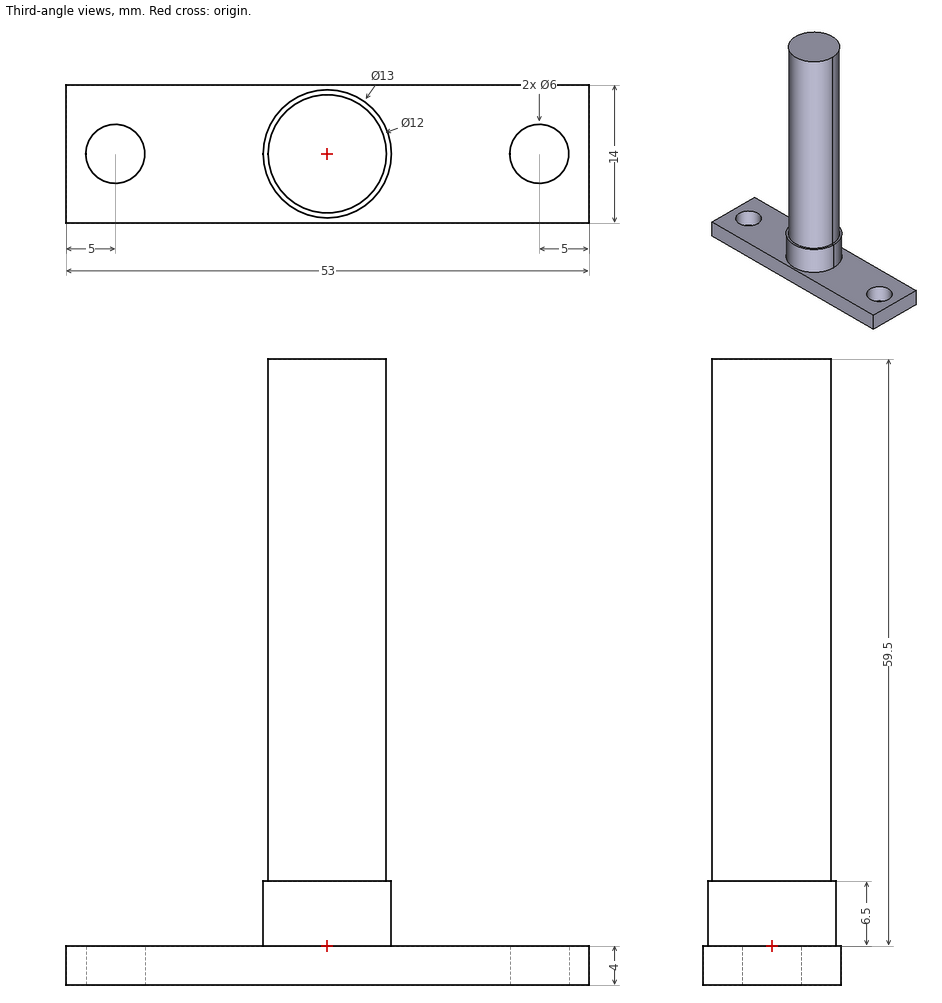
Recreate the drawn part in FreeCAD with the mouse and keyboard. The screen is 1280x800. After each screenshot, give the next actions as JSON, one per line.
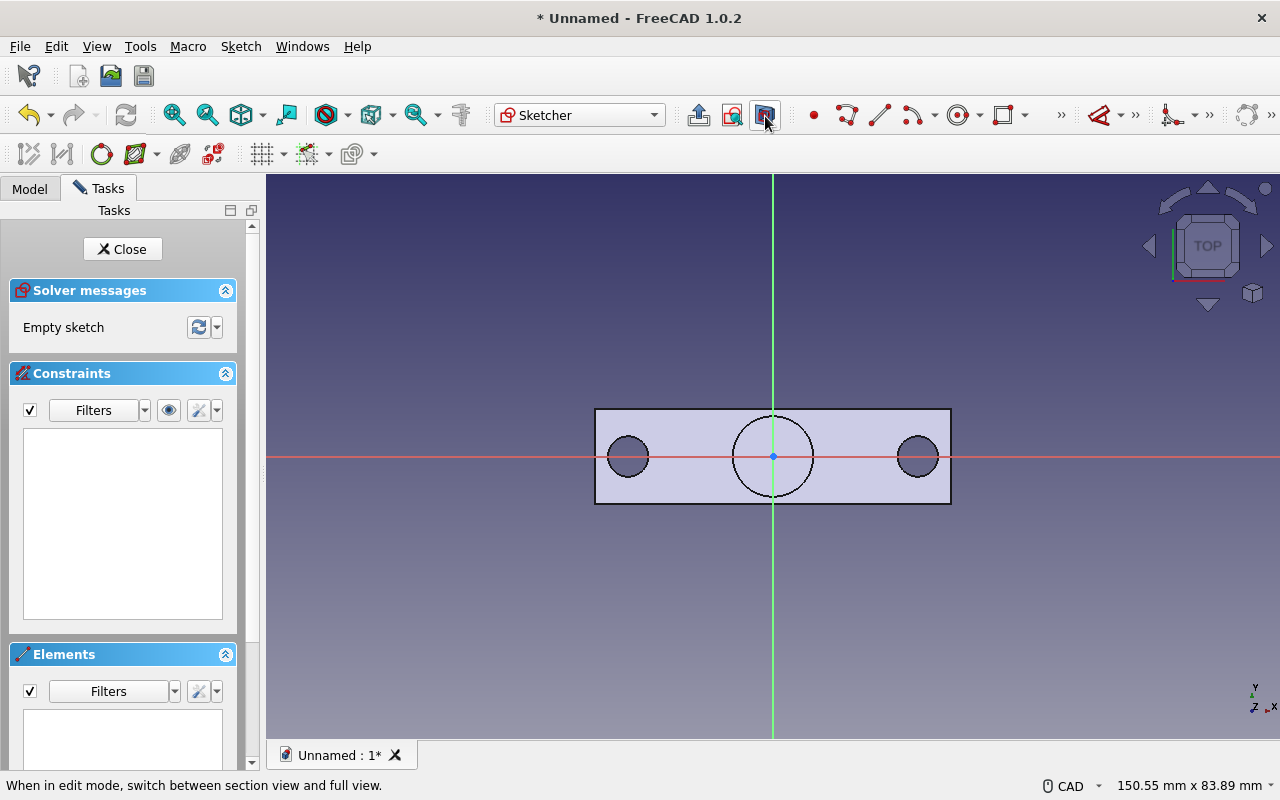
{"action": "scroll", "coordinate": [795, 456], "scroll_direction": "up", "scroll_amount": 7}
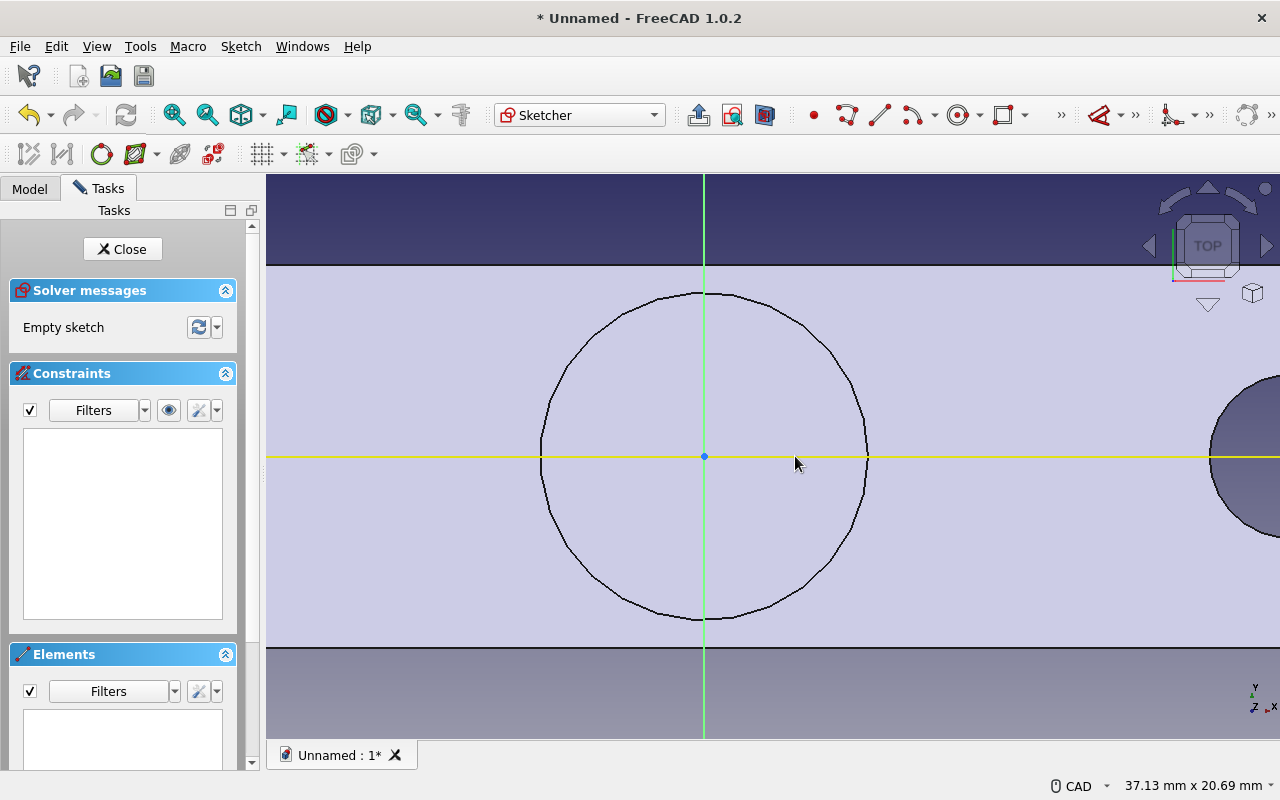
{"action": "key", "text": "g c"}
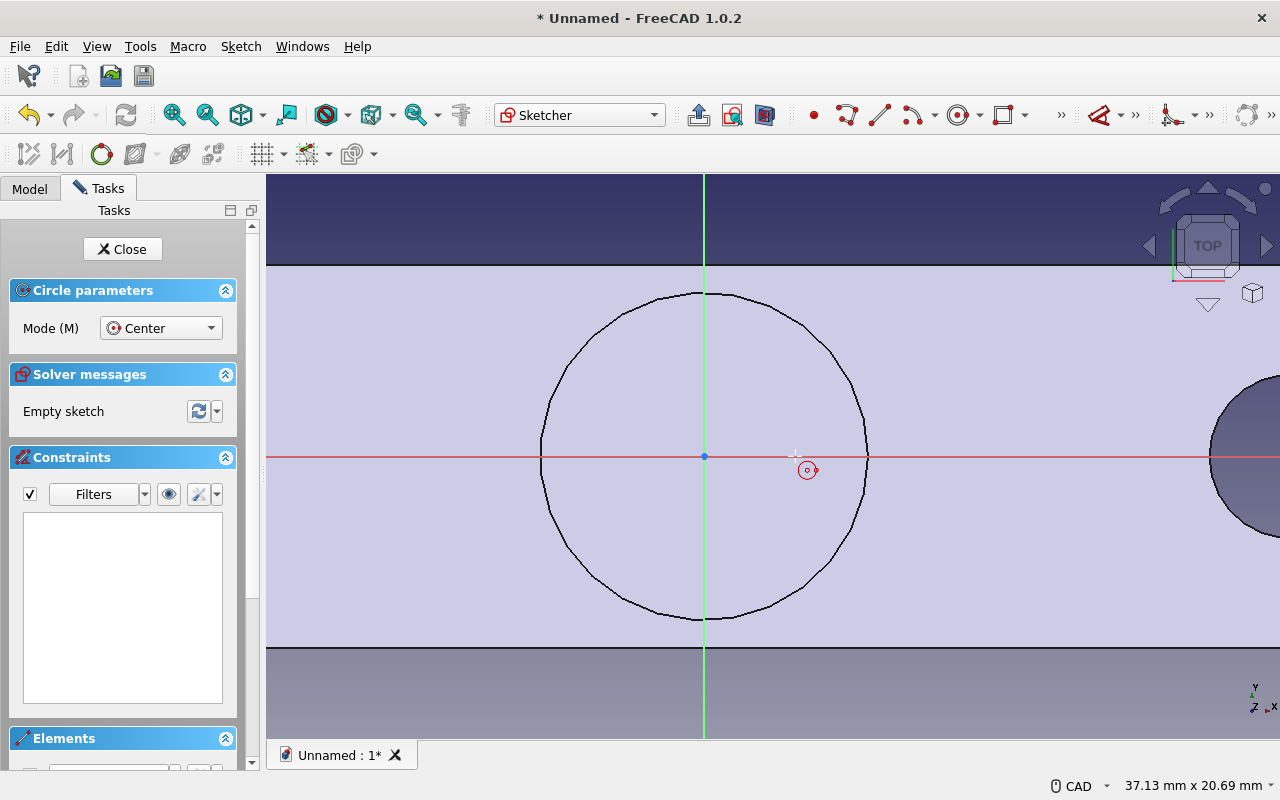
{"action": "left_click", "coordinate": [704, 456]}
{"action": "left_click", "coordinate": [830, 331]}
{"action": "key", "text": "Escape"}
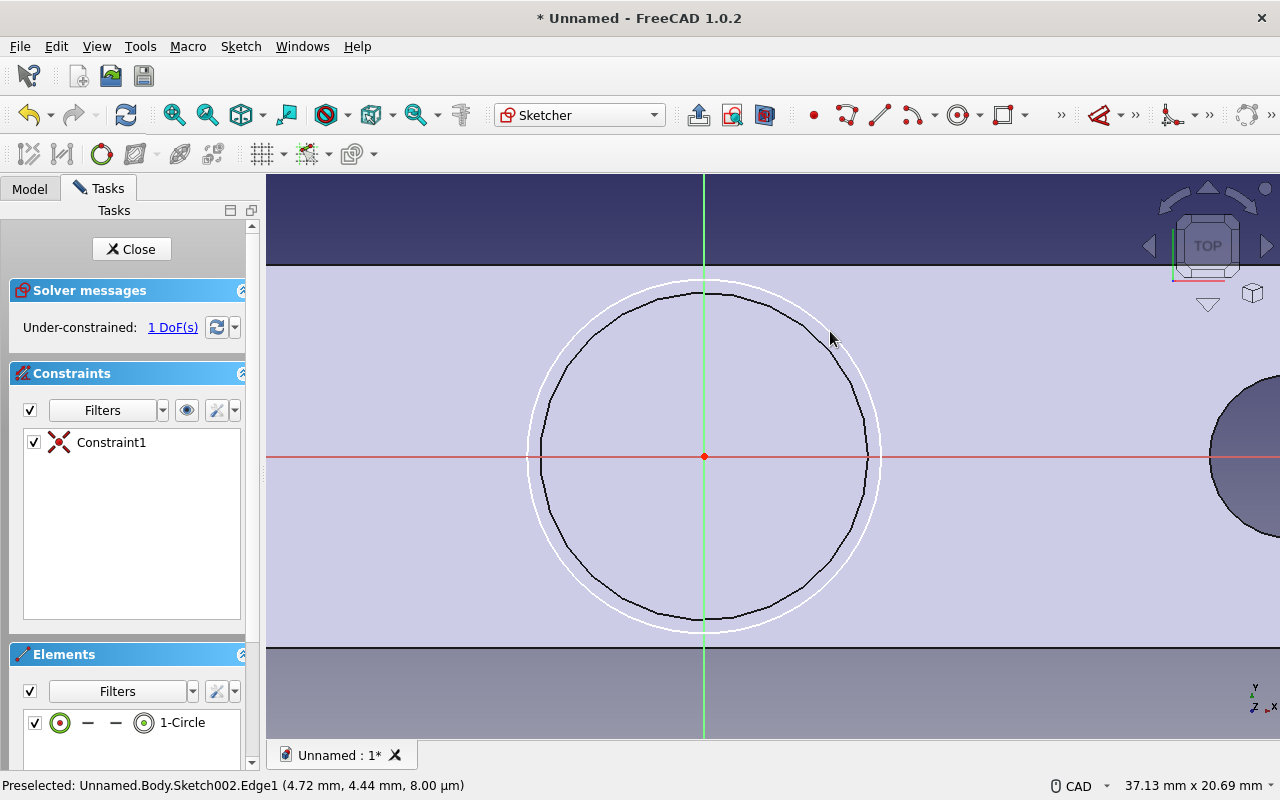
{"action": "key", "text": "d"}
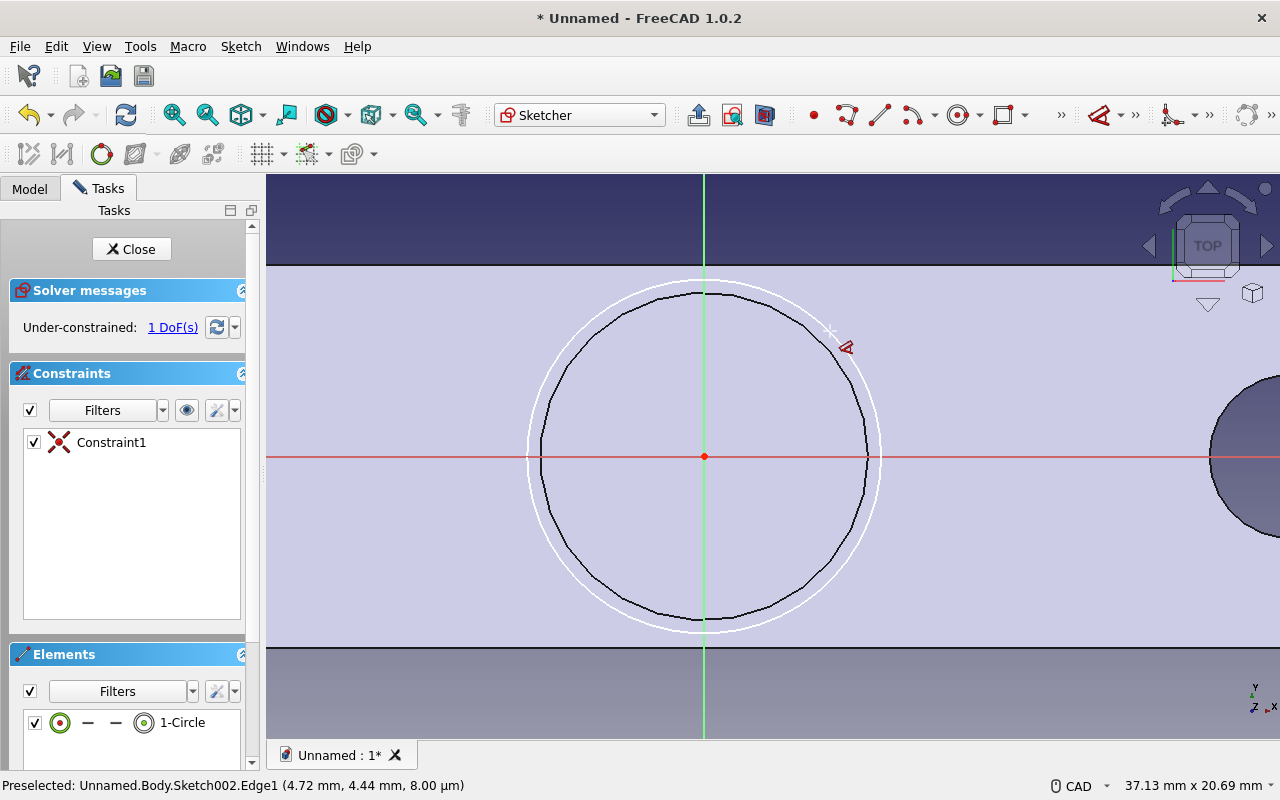
{"action": "left_click", "coordinate": [829, 331]}
{"action": "left_click", "coordinate": [852, 308]}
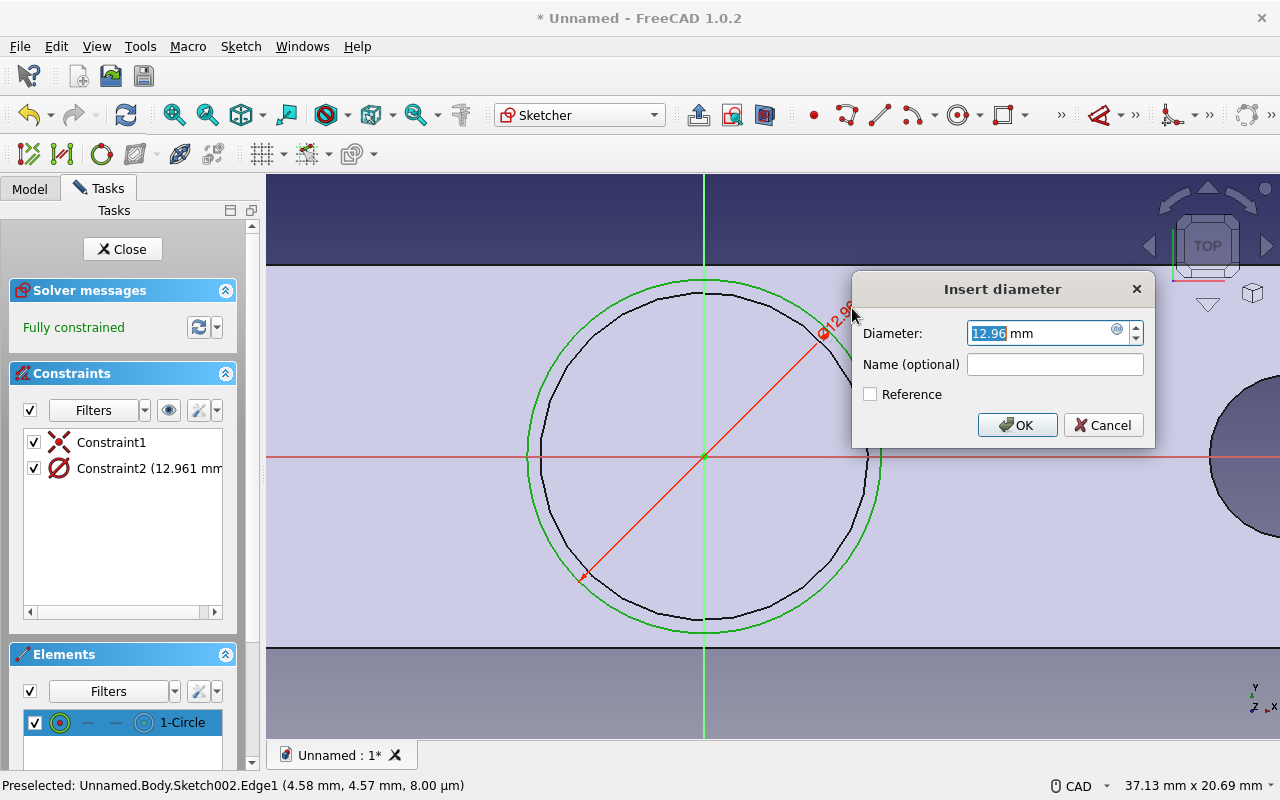
{"action": "type", "text": "13"}
{"action": "key", "text": "Return"}
{"action": "key", "text": "Escape"}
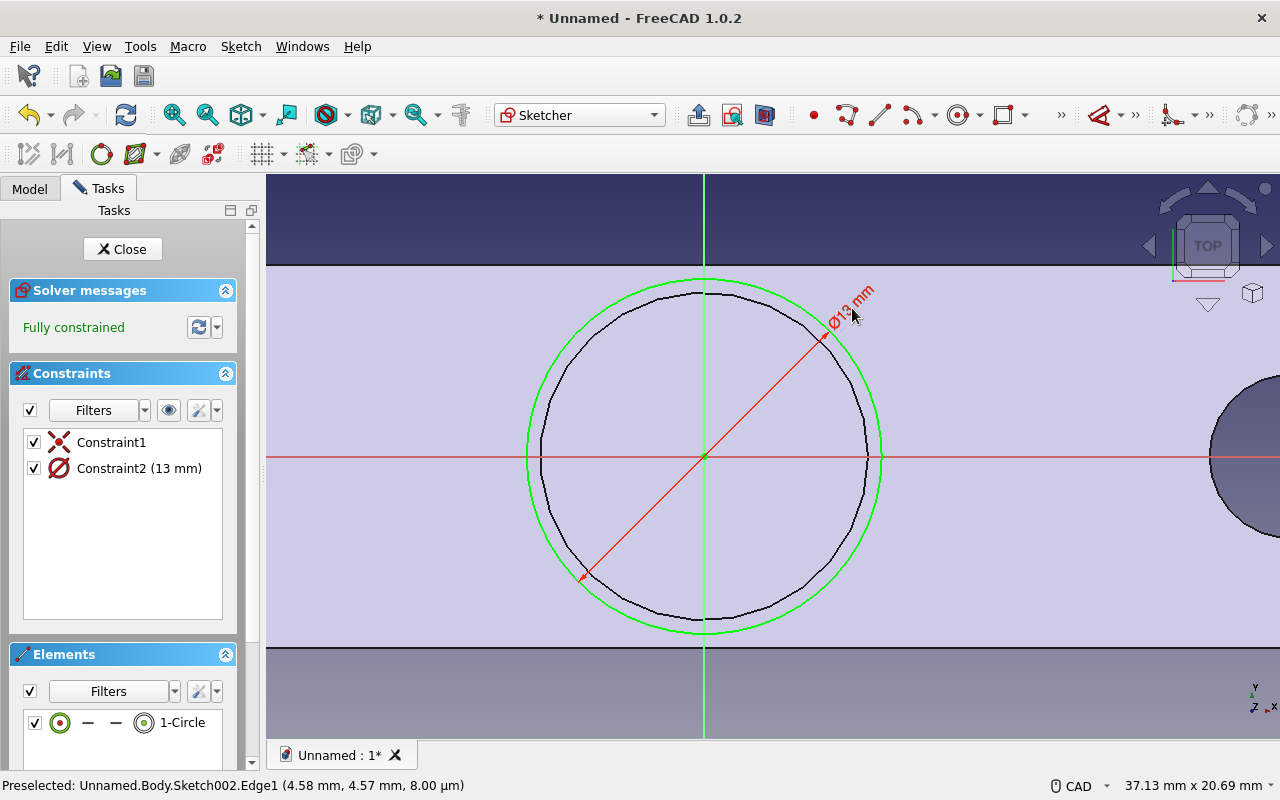
{"action": "left_click", "coordinate": [123, 249]}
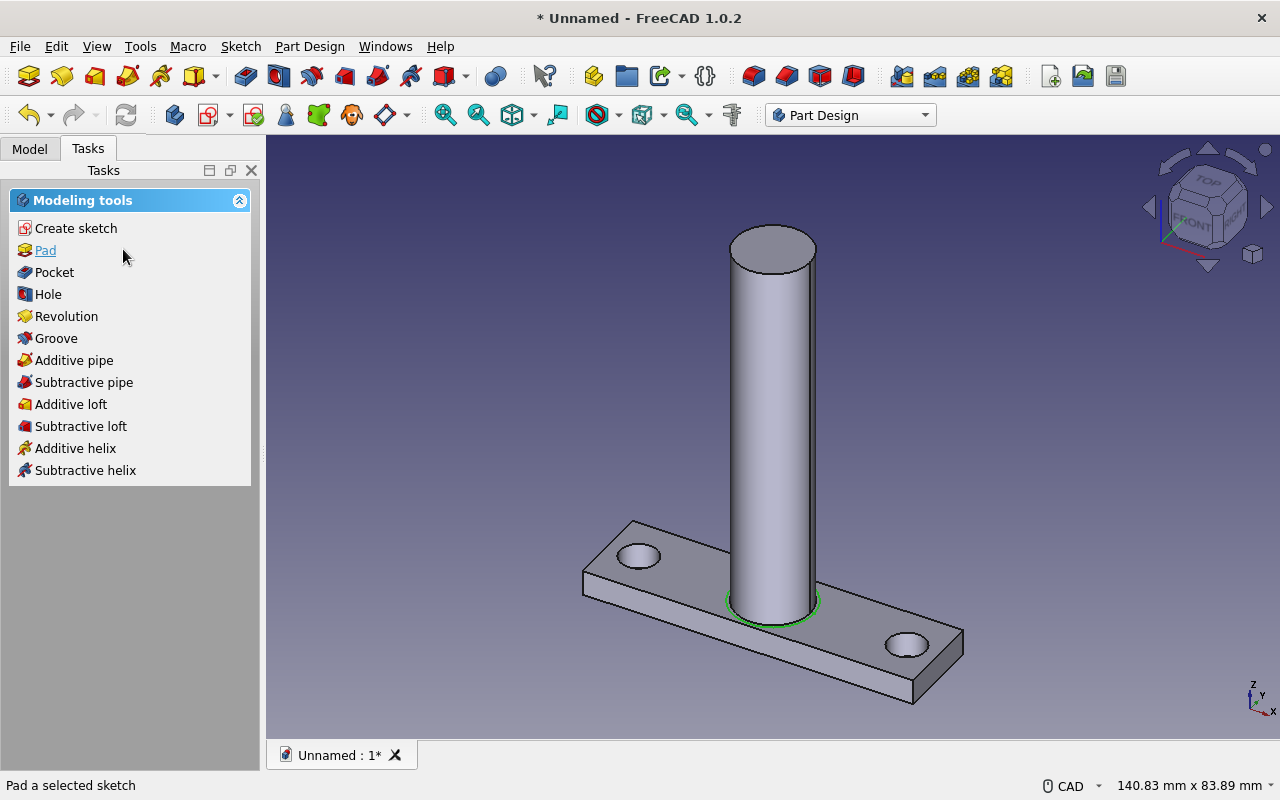
{"action": "left_click", "coordinate": [29, 76]}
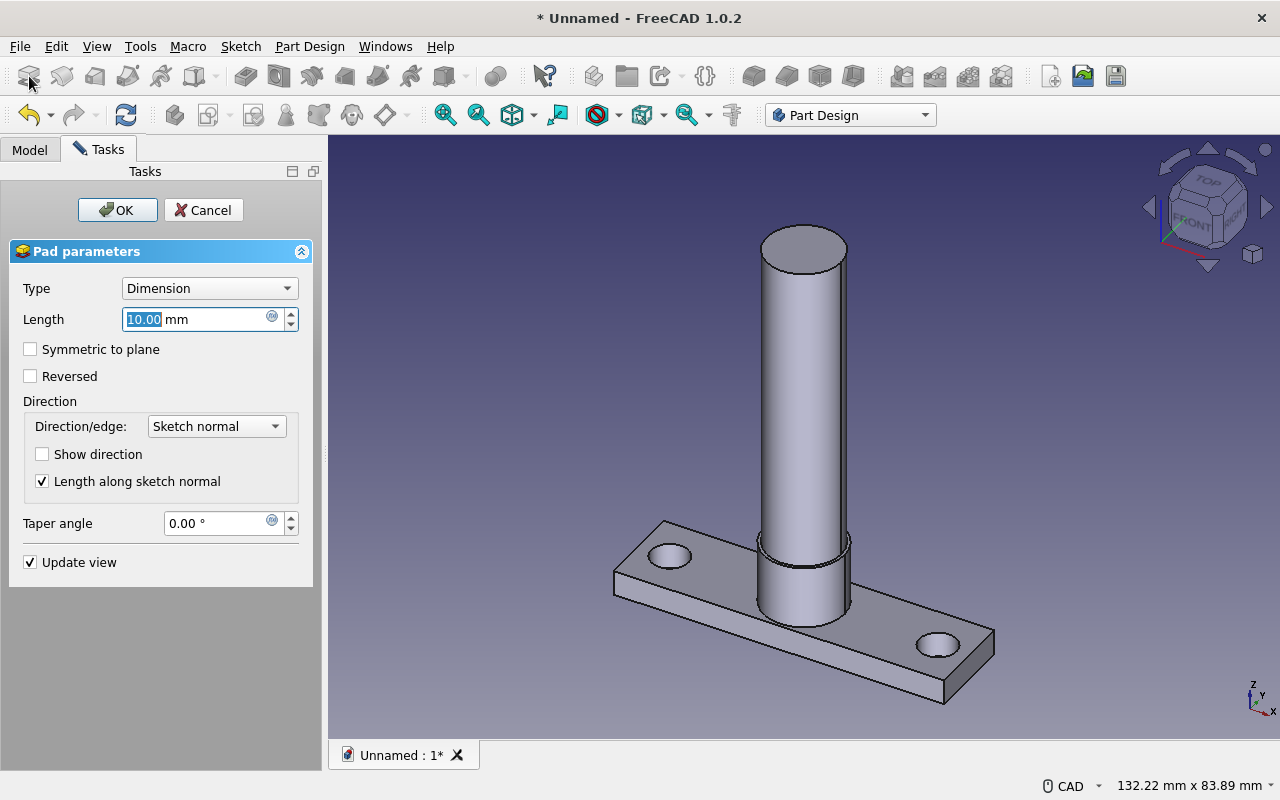
{"action": "type", "text": "6.5"}
{"action": "key", "text": "Tab"}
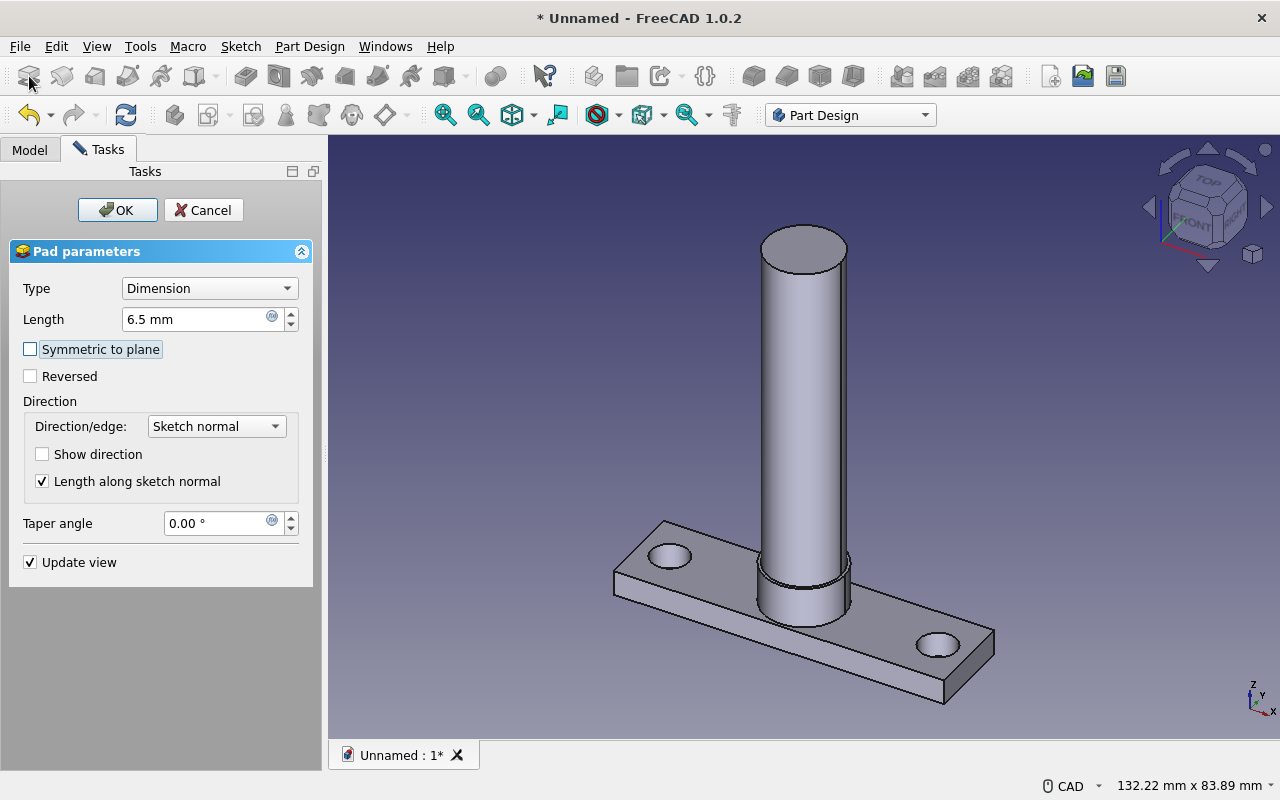
{"action": "left_click", "coordinate": [118, 210]}